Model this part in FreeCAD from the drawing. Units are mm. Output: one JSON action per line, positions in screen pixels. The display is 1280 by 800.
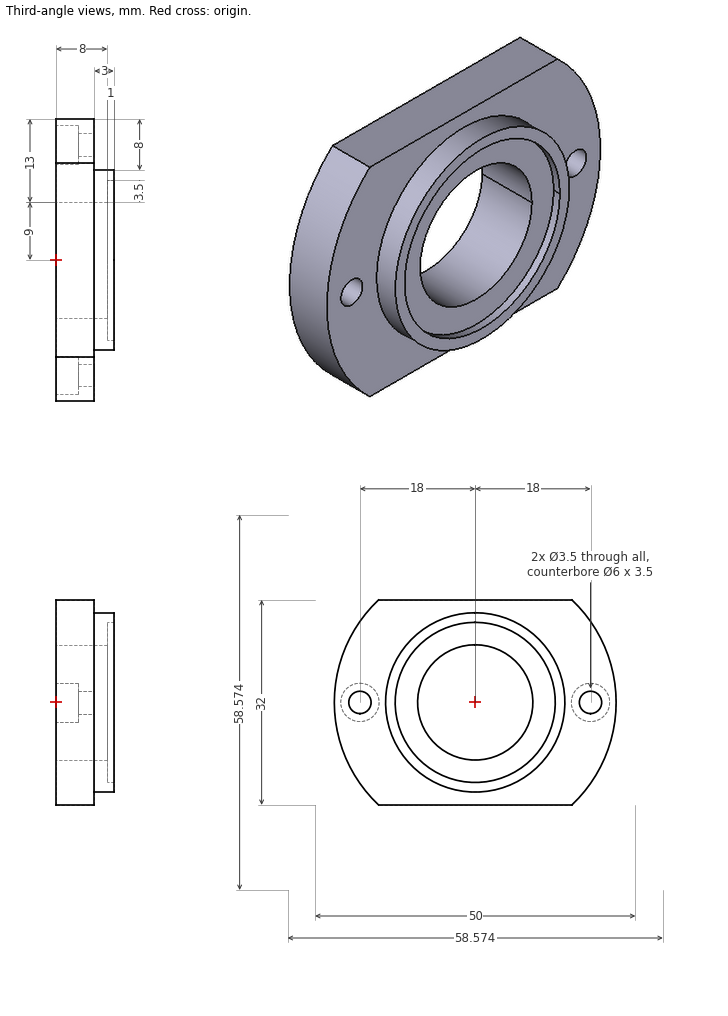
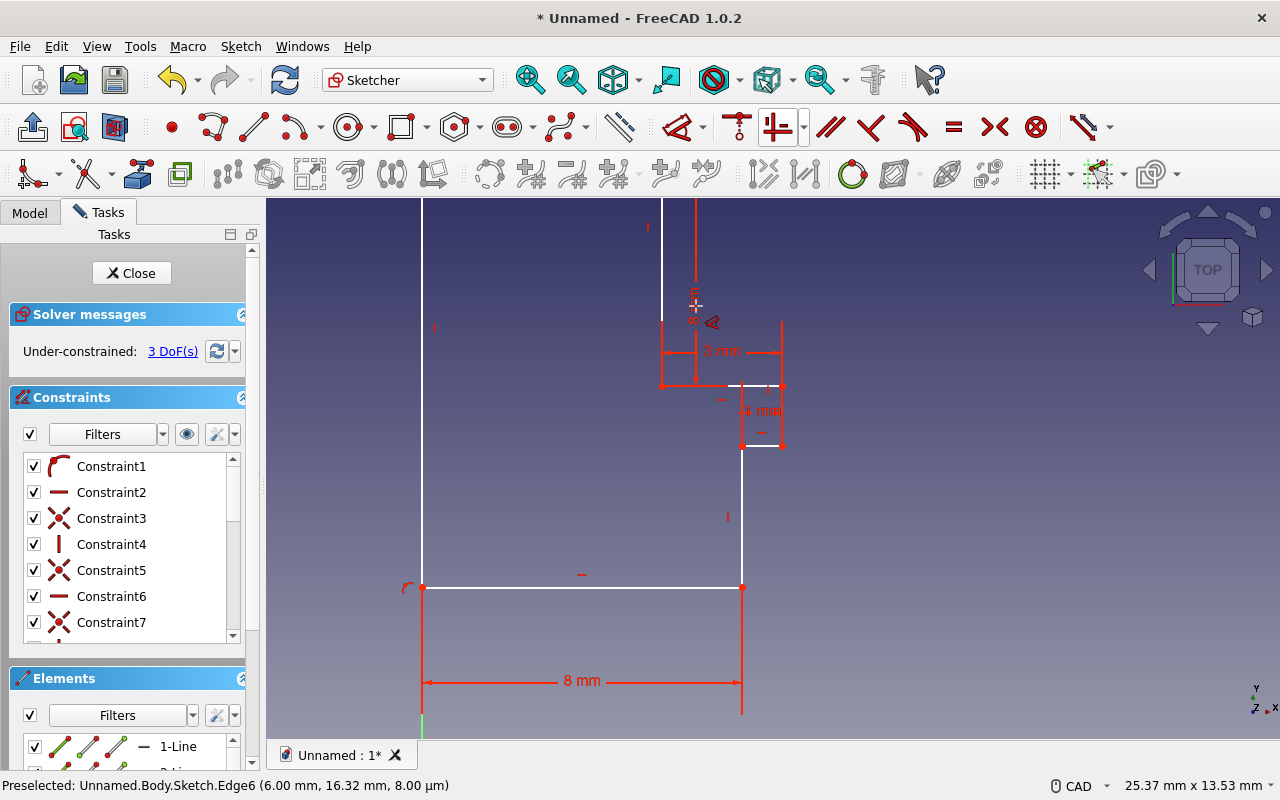
{"action": "left_click", "coordinate": [422, 431]}
{"action": "left_click", "coordinate": [388, 407]}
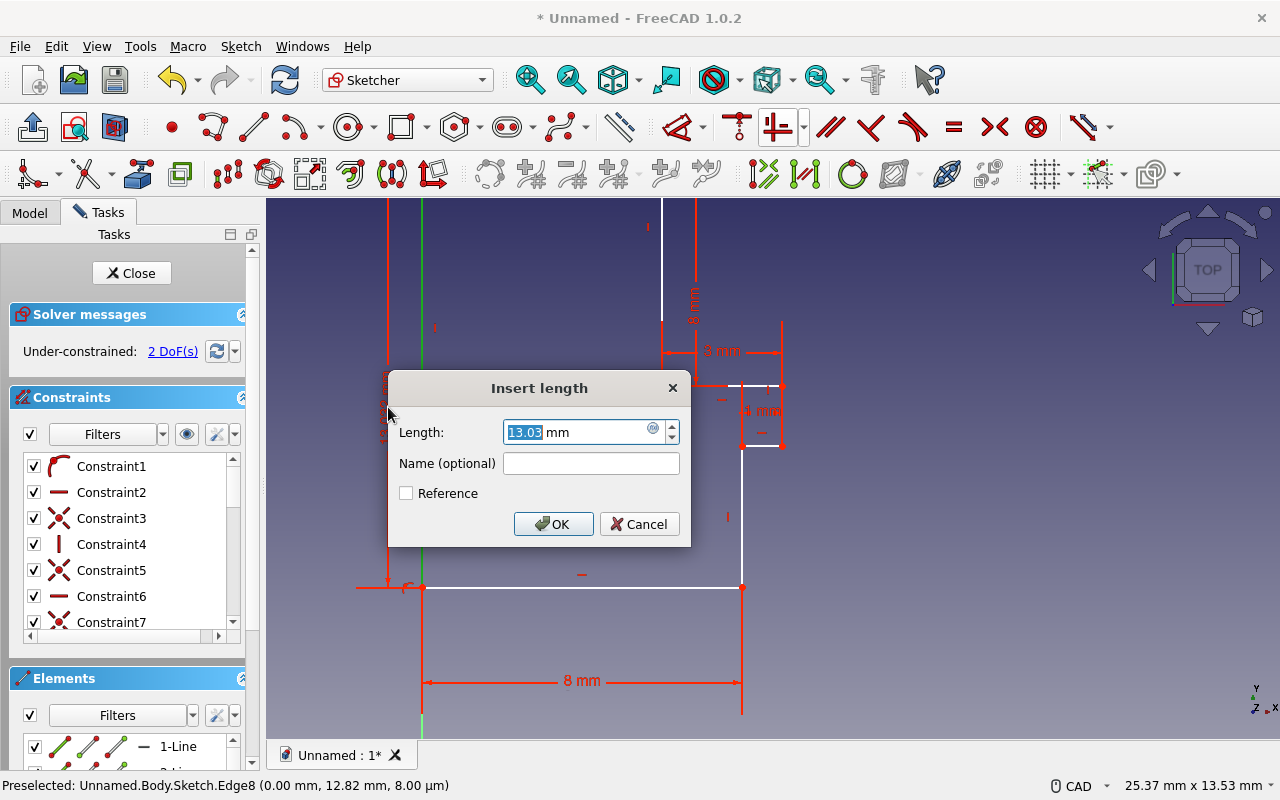
{"action": "type", "text": "13"}
{"action": "key", "text": "Return"}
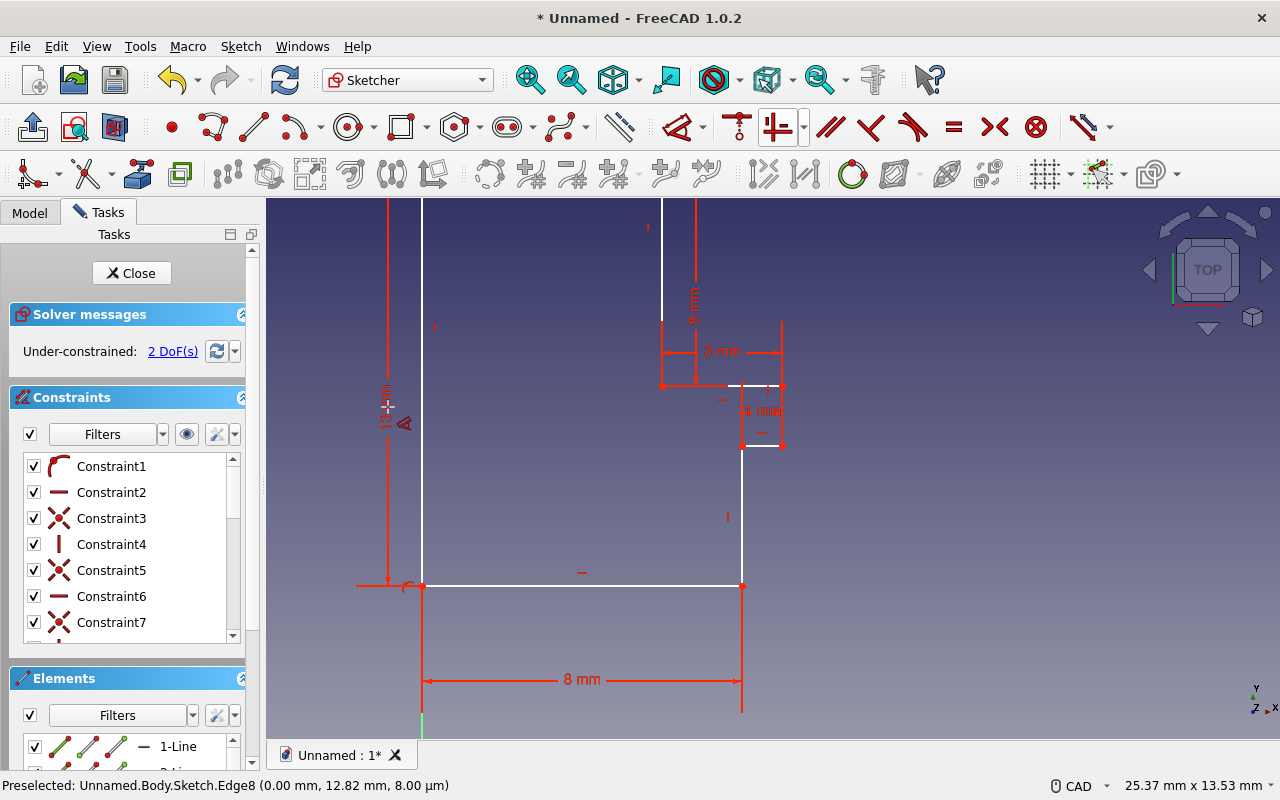
{"action": "left_click", "coordinate": [422, 586]}
{"action": "left_click", "coordinate": [388, 649]}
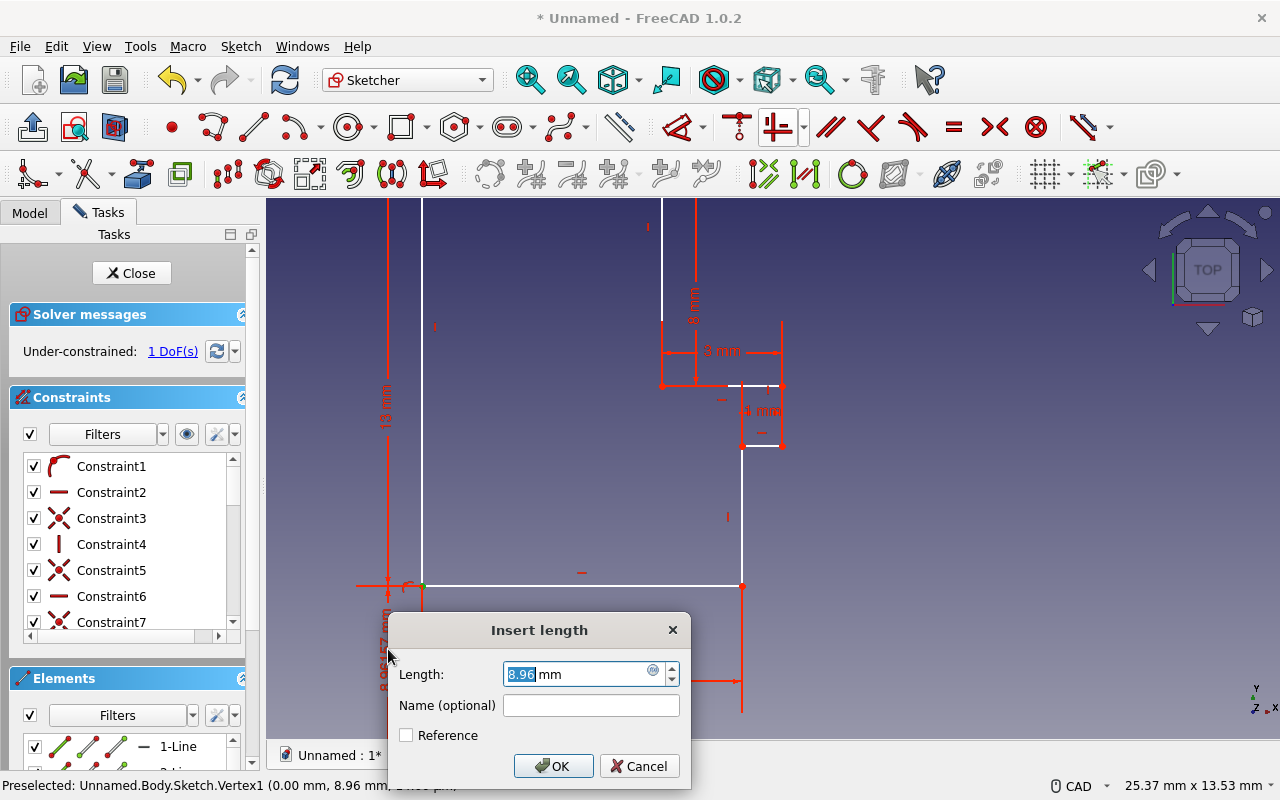
{"action": "type", "text": "9"}
{"action": "key", "text": "Return"}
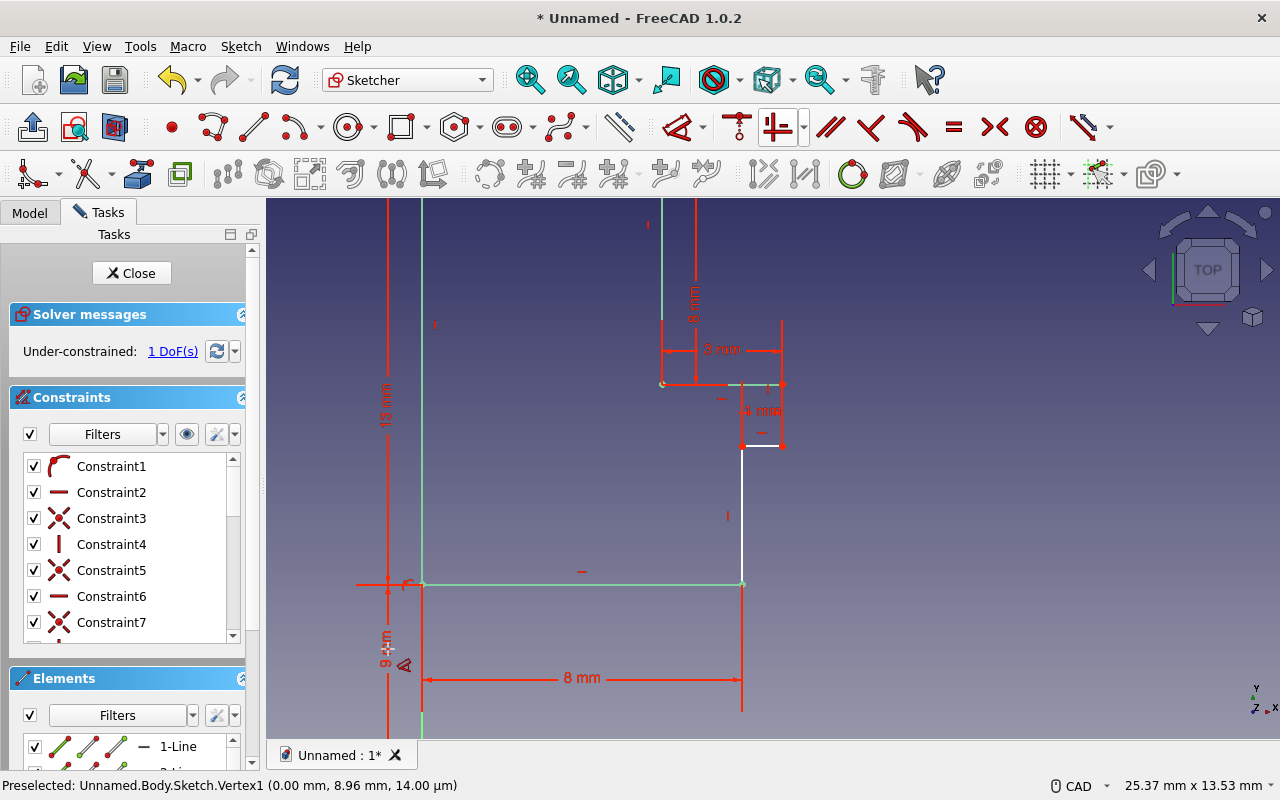
{"action": "left_click", "coordinate": [742, 543]}
{"action": "left_click", "coordinate": [776, 515]}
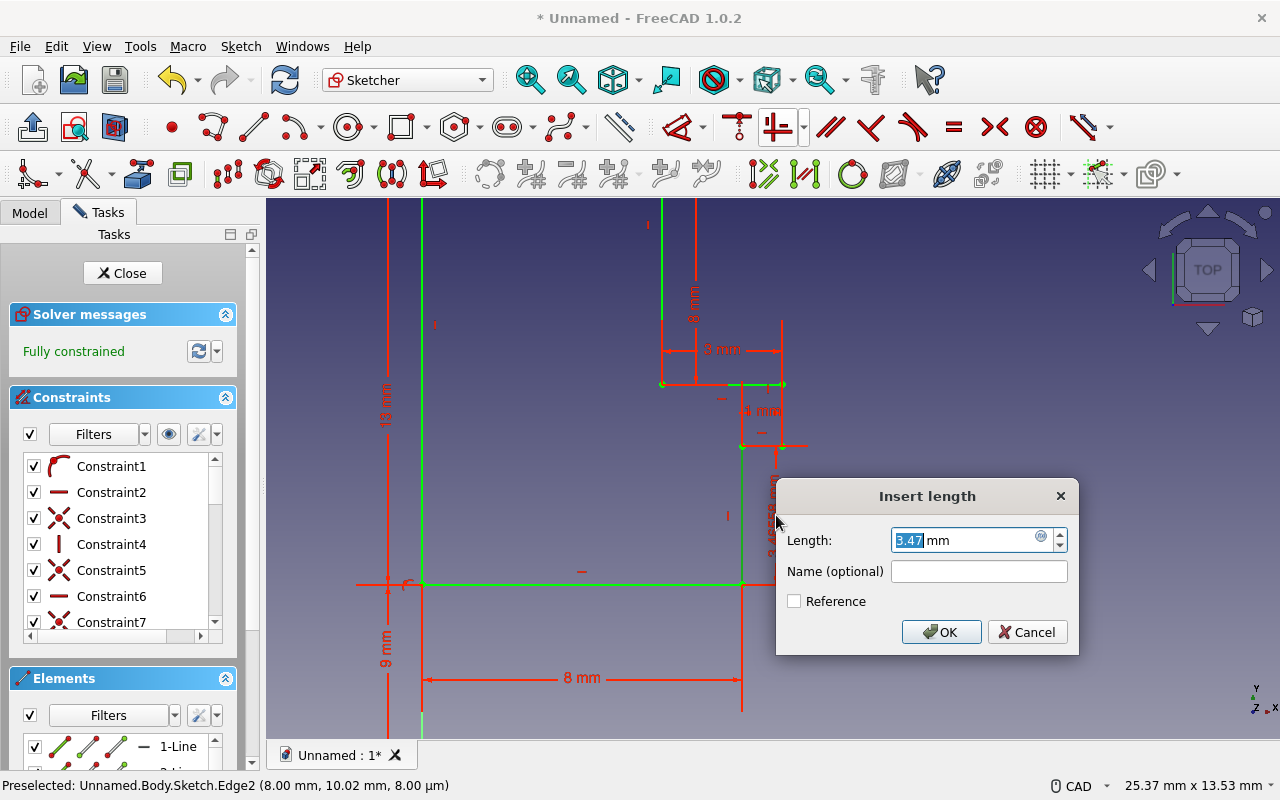
{"action": "type", "text": "3.5"}
{"action": "key", "text": "Return"}
{"action": "key", "text": "Escape"}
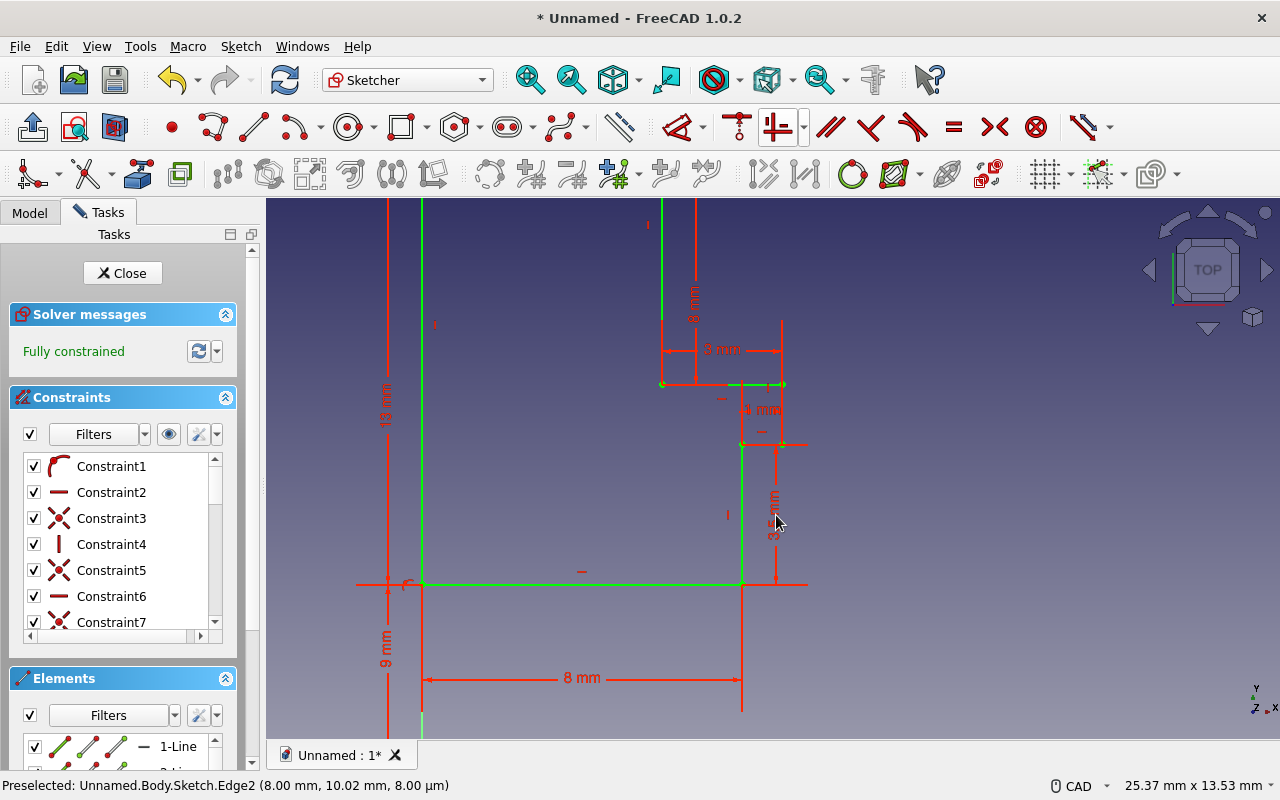
{"action": "left_click", "coordinate": [123, 273]}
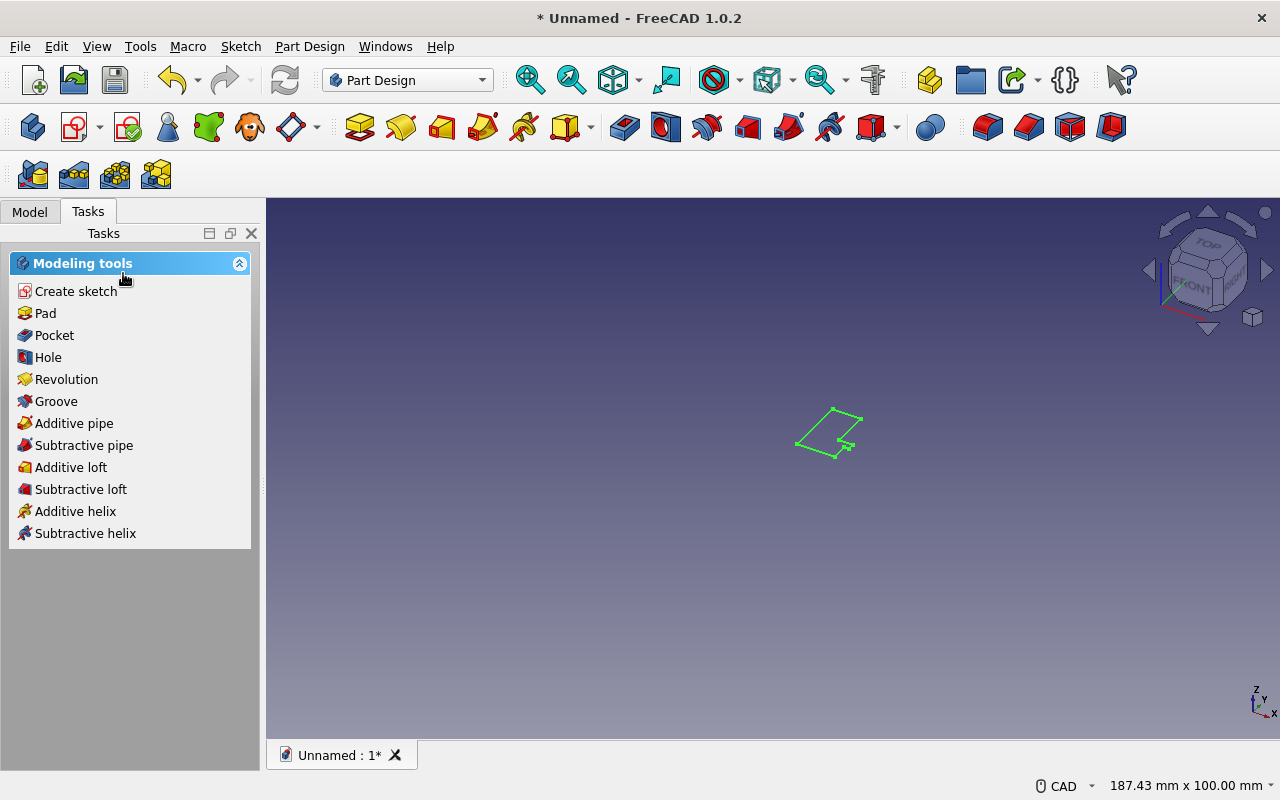
{"action": "left_click", "coordinate": [401, 128]}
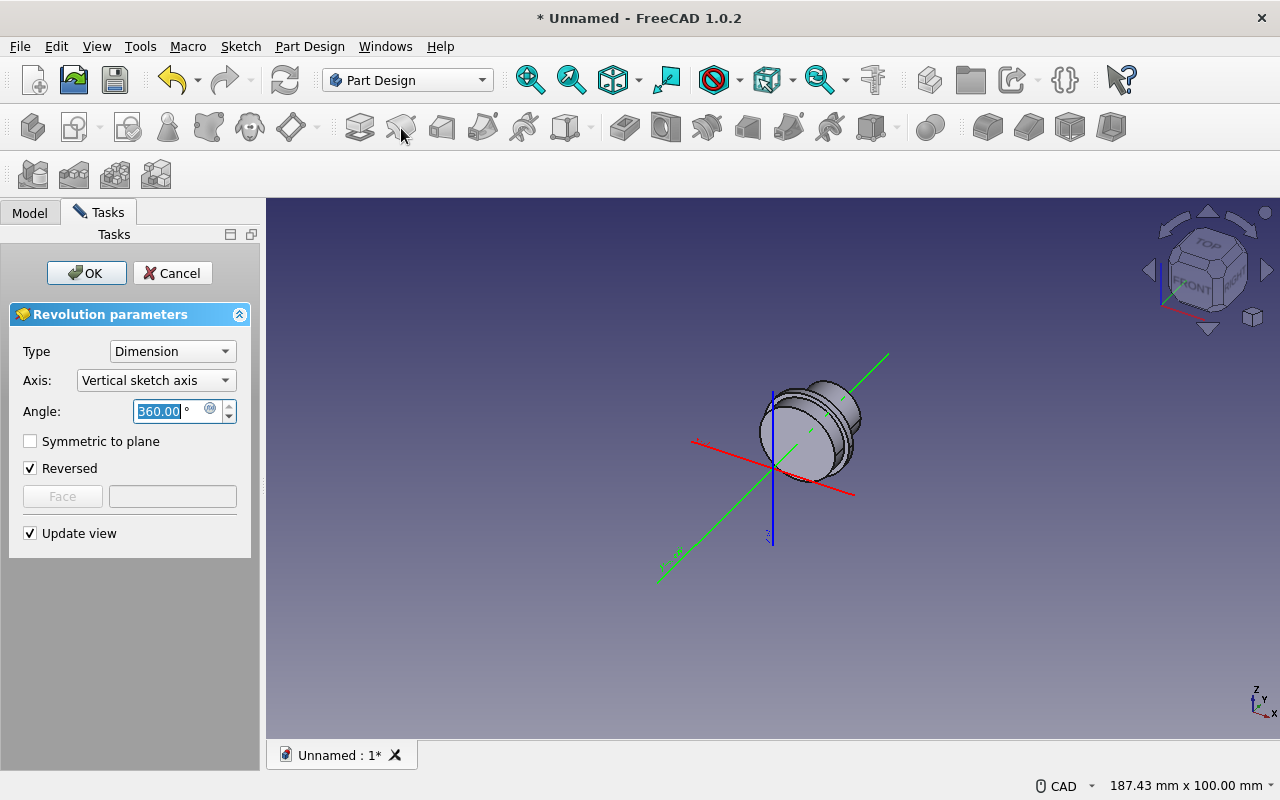
{"action": "left_click", "coordinate": [157, 380]}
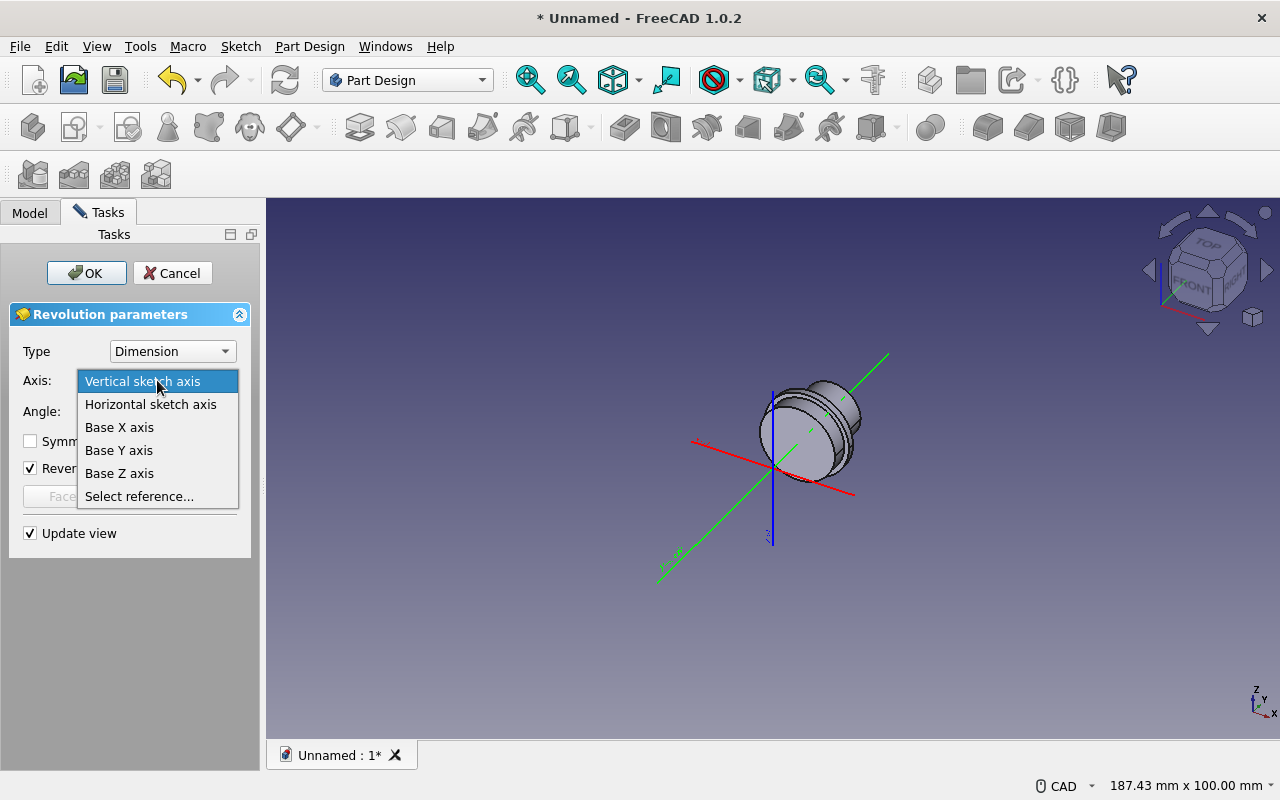
{"action": "left_click", "coordinate": [156, 404]}